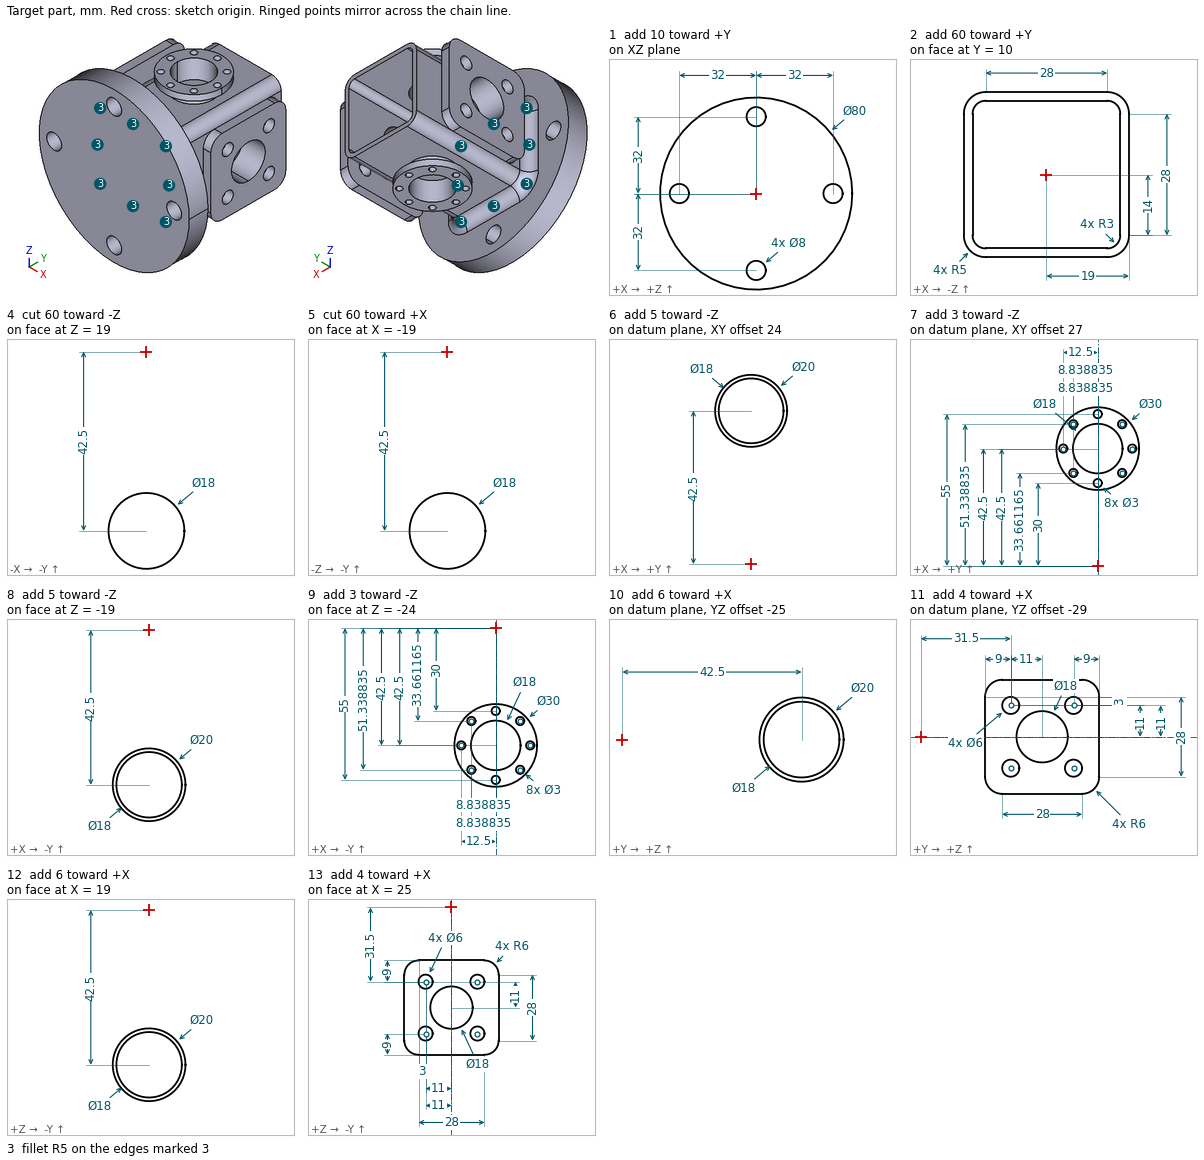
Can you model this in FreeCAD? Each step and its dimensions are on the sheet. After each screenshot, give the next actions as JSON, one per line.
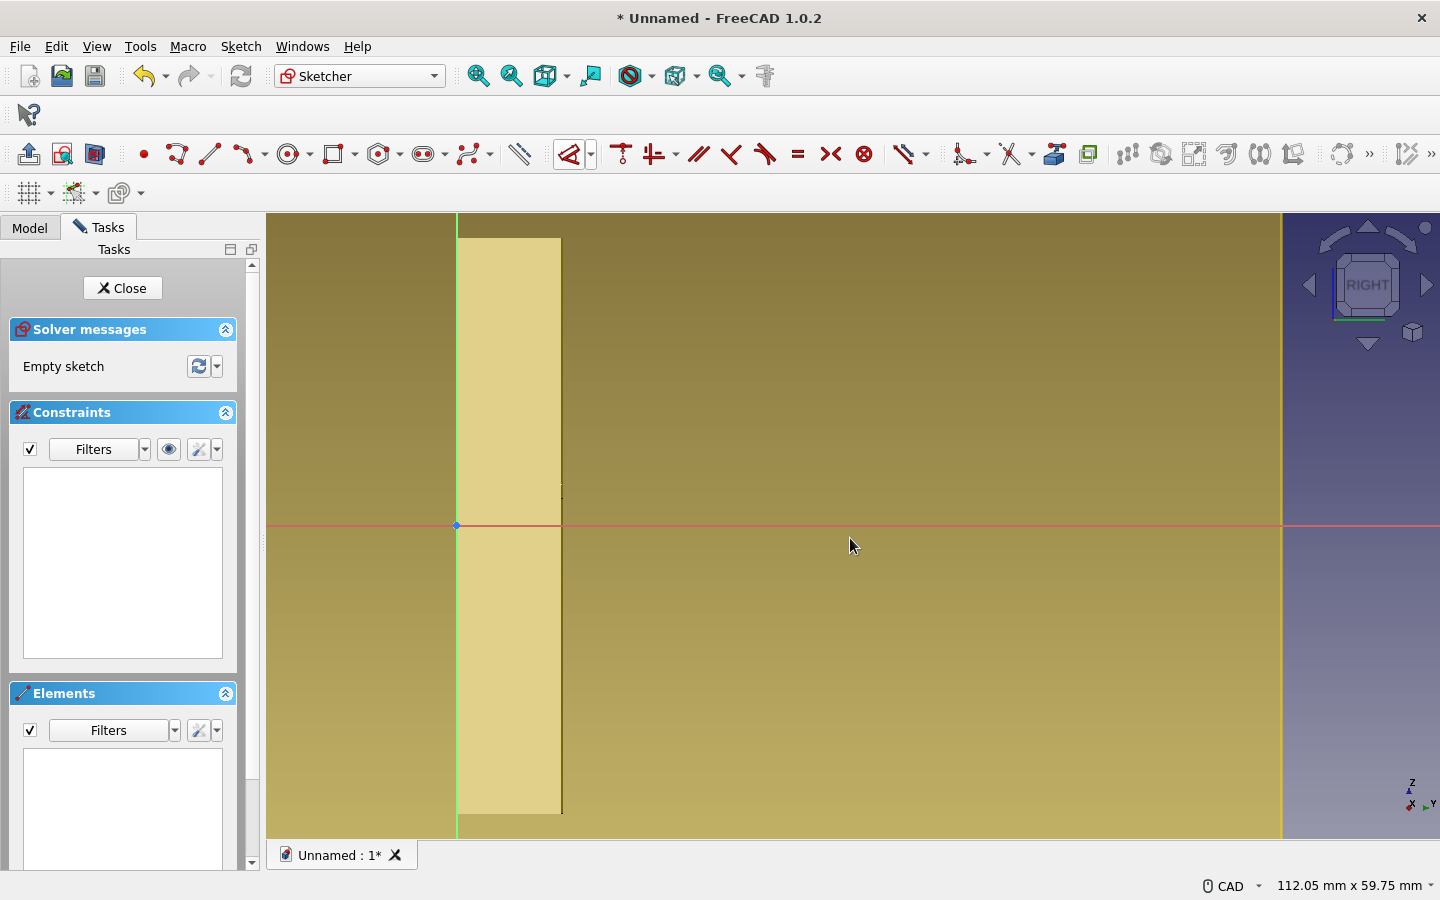
{"action": "key", "text": "g l"}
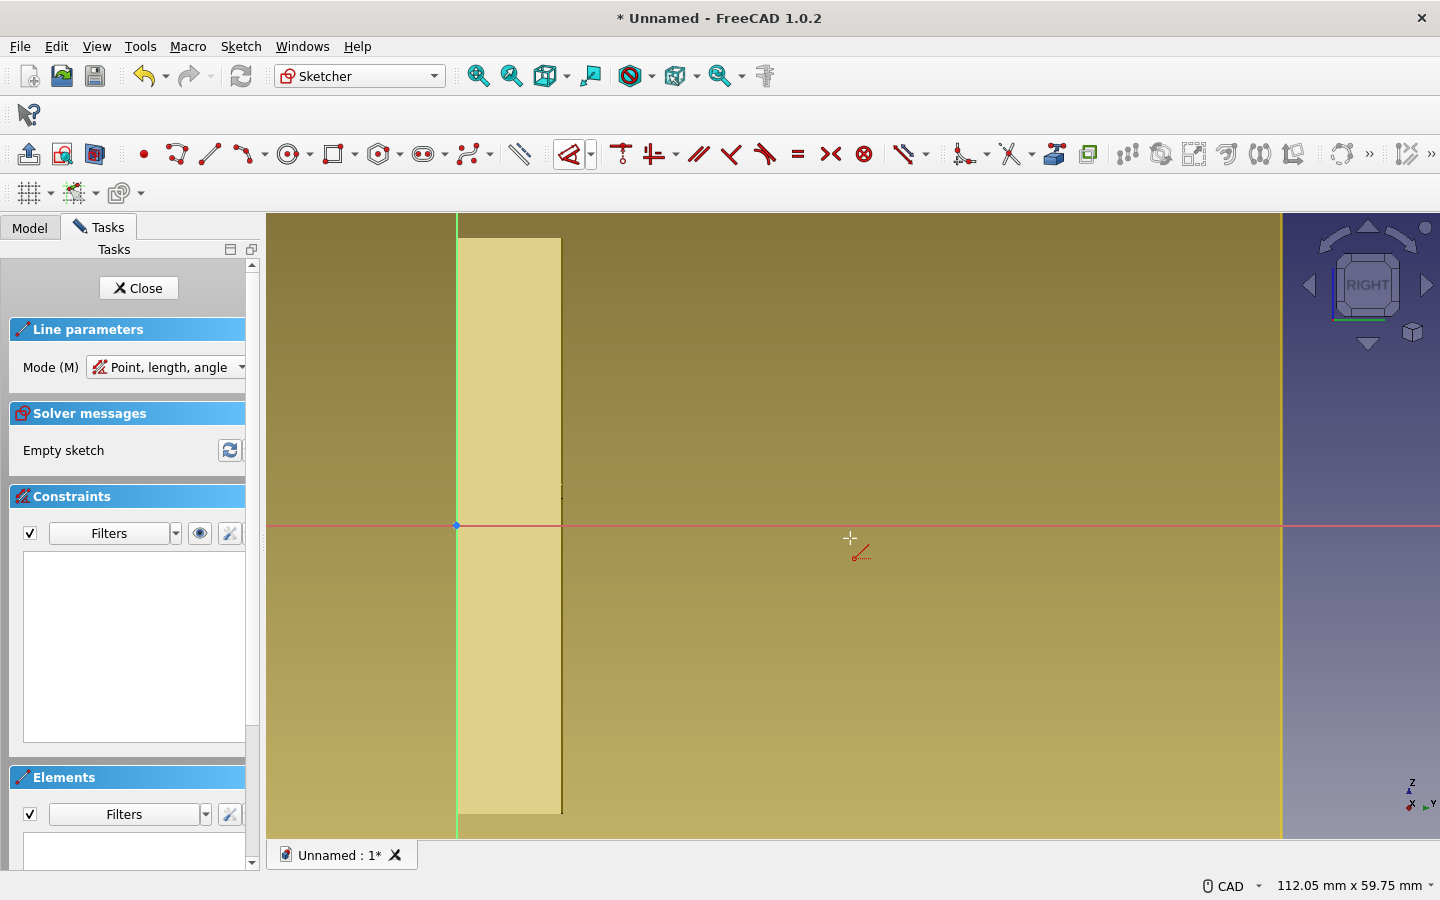
{"action": "left_click", "coordinate": [1112, 379]}
{"action": "left_click", "coordinate": [1112, 673]}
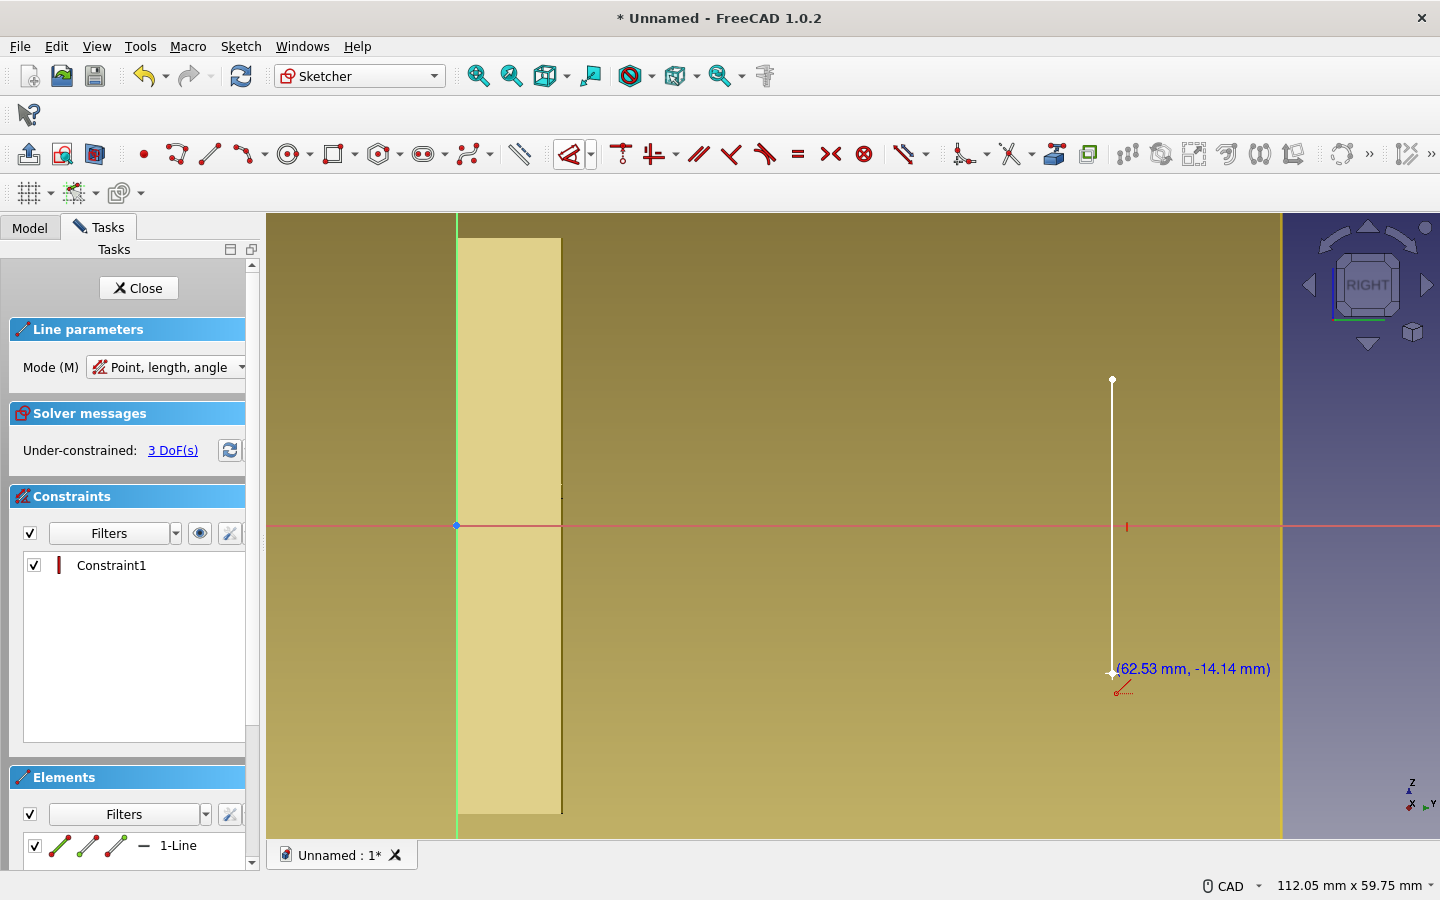
{"action": "left_click", "coordinate": [1049, 735]}
{"action": "left_click", "coordinate": [755, 735]}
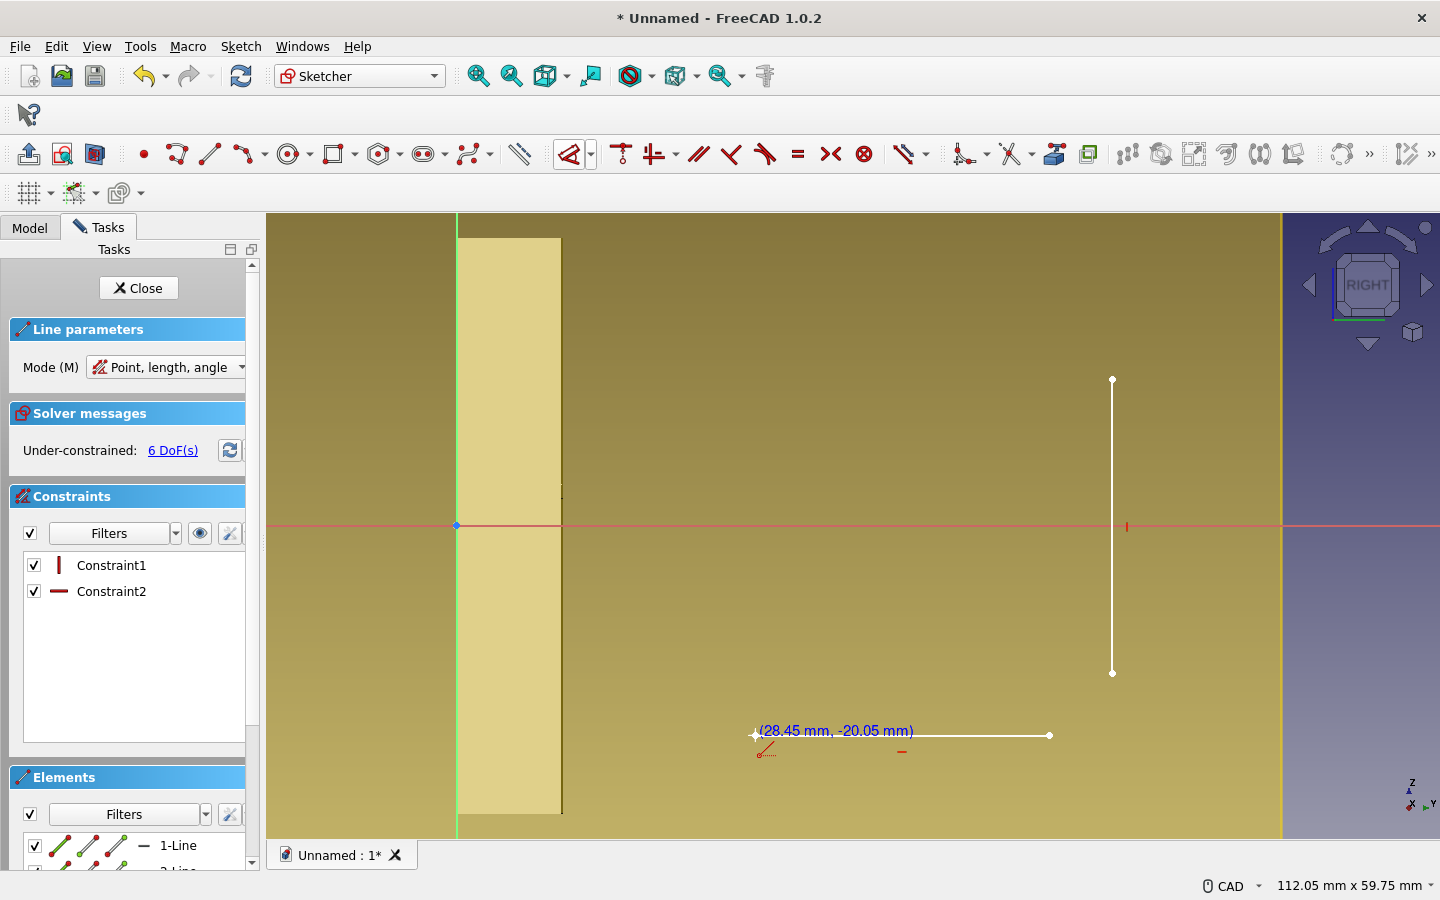
{"action": "left_click", "coordinate": [693, 673]}
{"action": "left_click", "coordinate": [693, 379]}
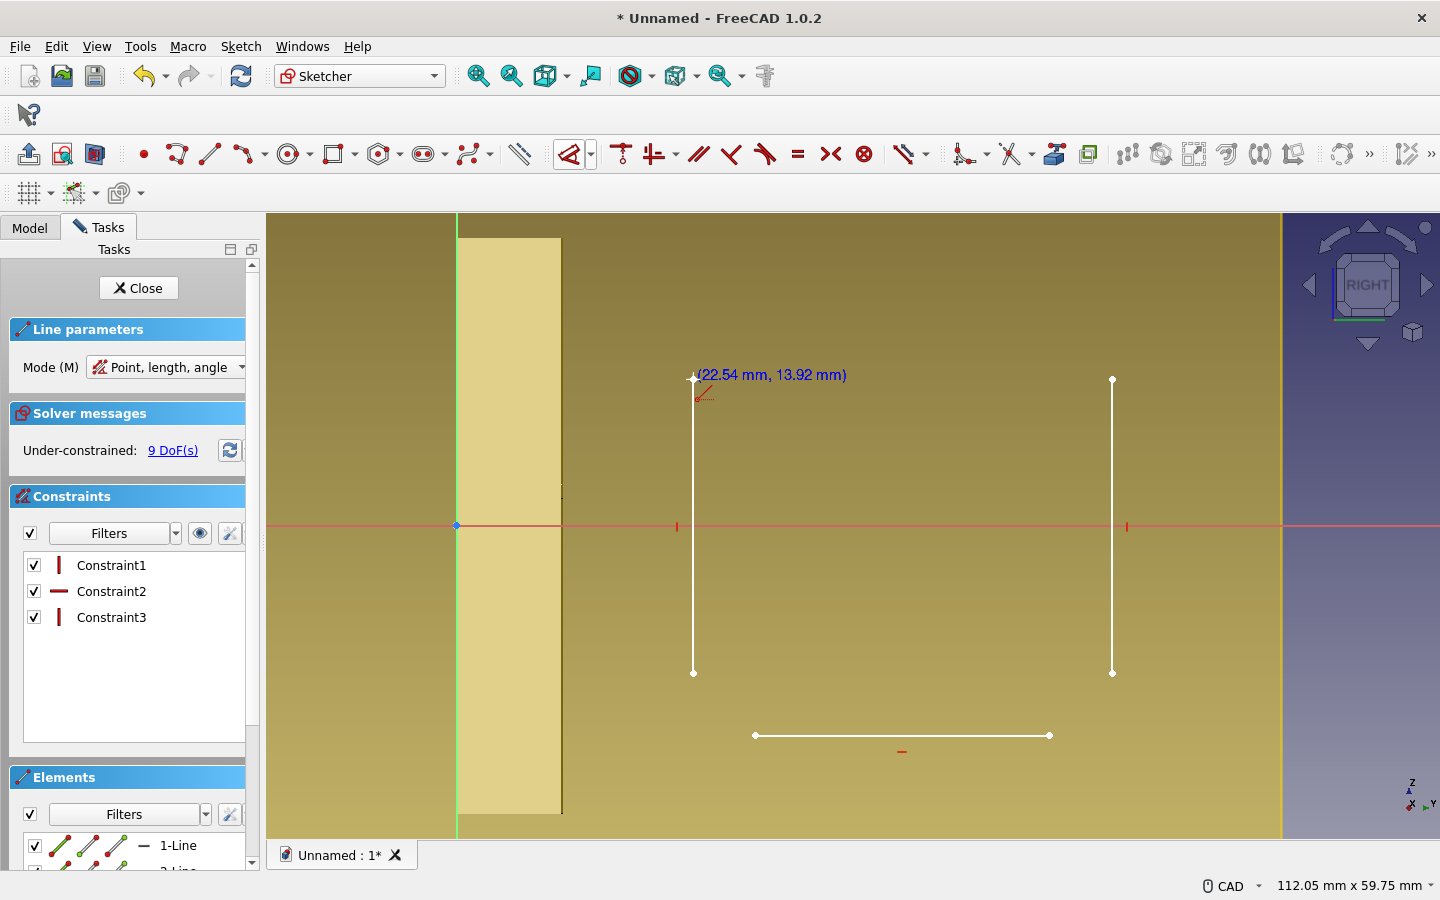
{"action": "left_click", "coordinate": [755, 316]}
{"action": "left_click", "coordinate": [1049, 316]}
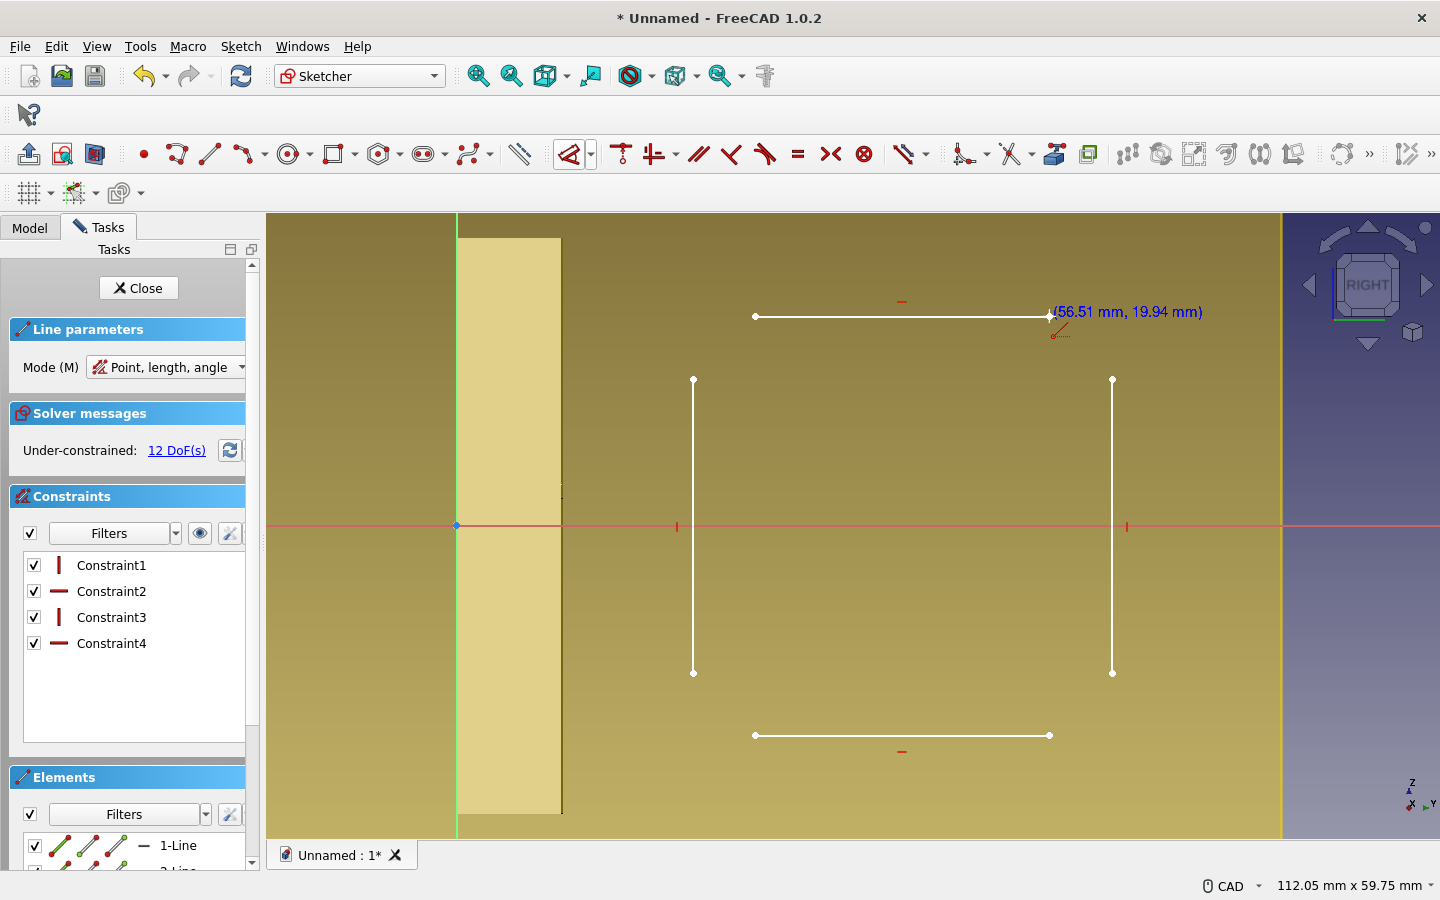
{"action": "key", "text": "g 3 a"}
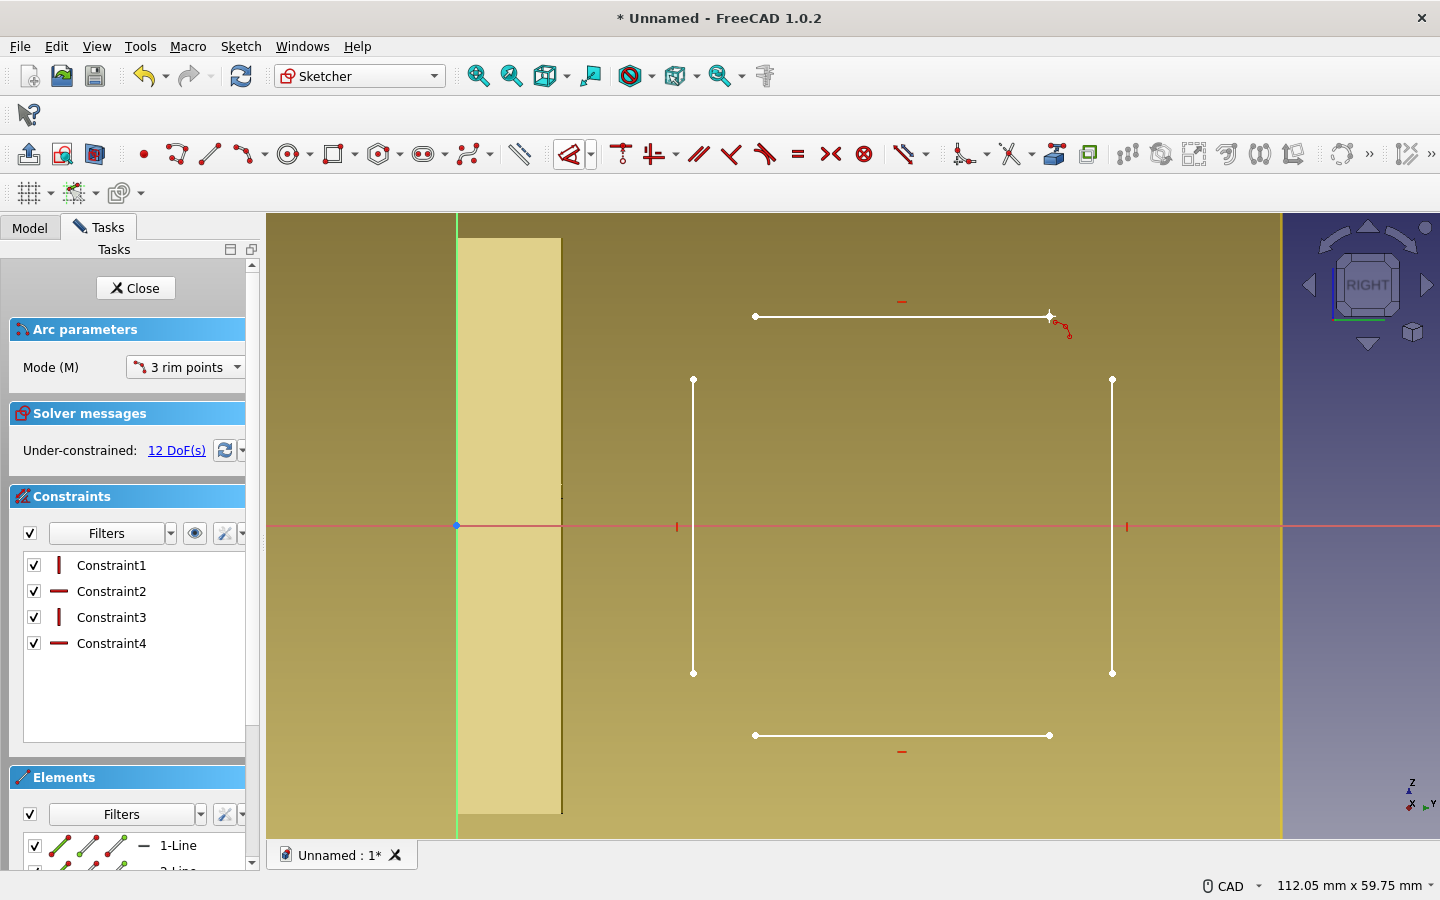
{"action": "left_click", "coordinate": [1112, 674]}
{"action": "left_click", "coordinate": [1049, 736]}
{"action": "left_click", "coordinate": [1093, 717]}